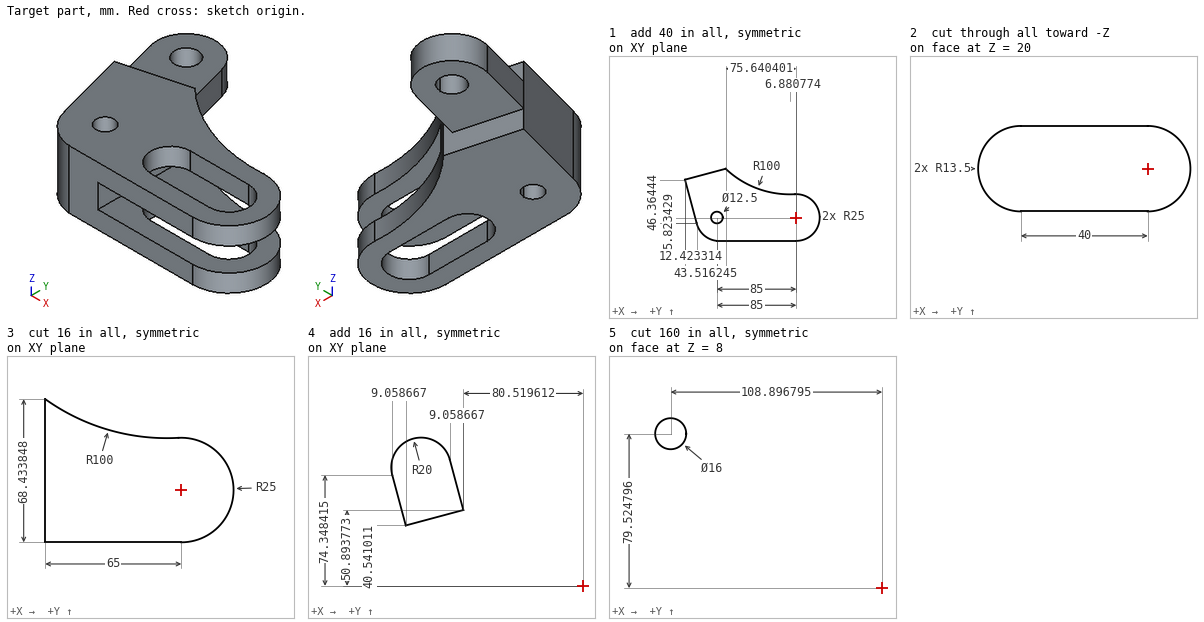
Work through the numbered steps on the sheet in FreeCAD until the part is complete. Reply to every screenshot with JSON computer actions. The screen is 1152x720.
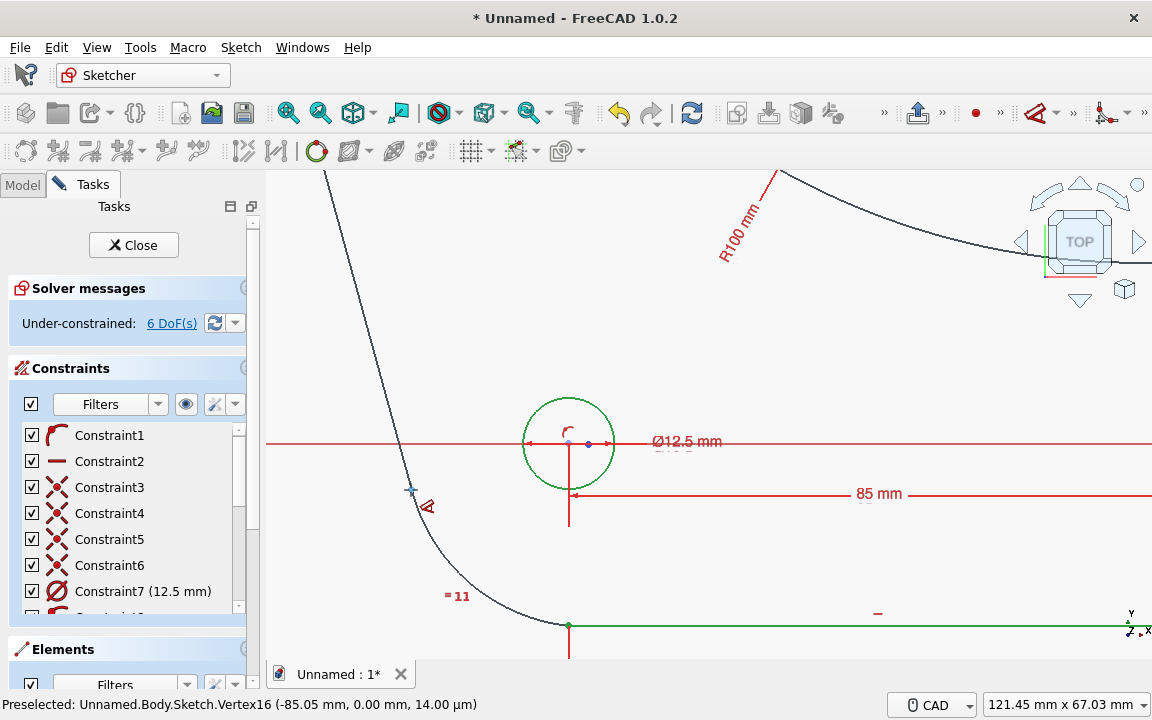
{"action": "left_click", "coordinate": [412, 489]}
{"action": "left_click", "coordinate": [378, 466]}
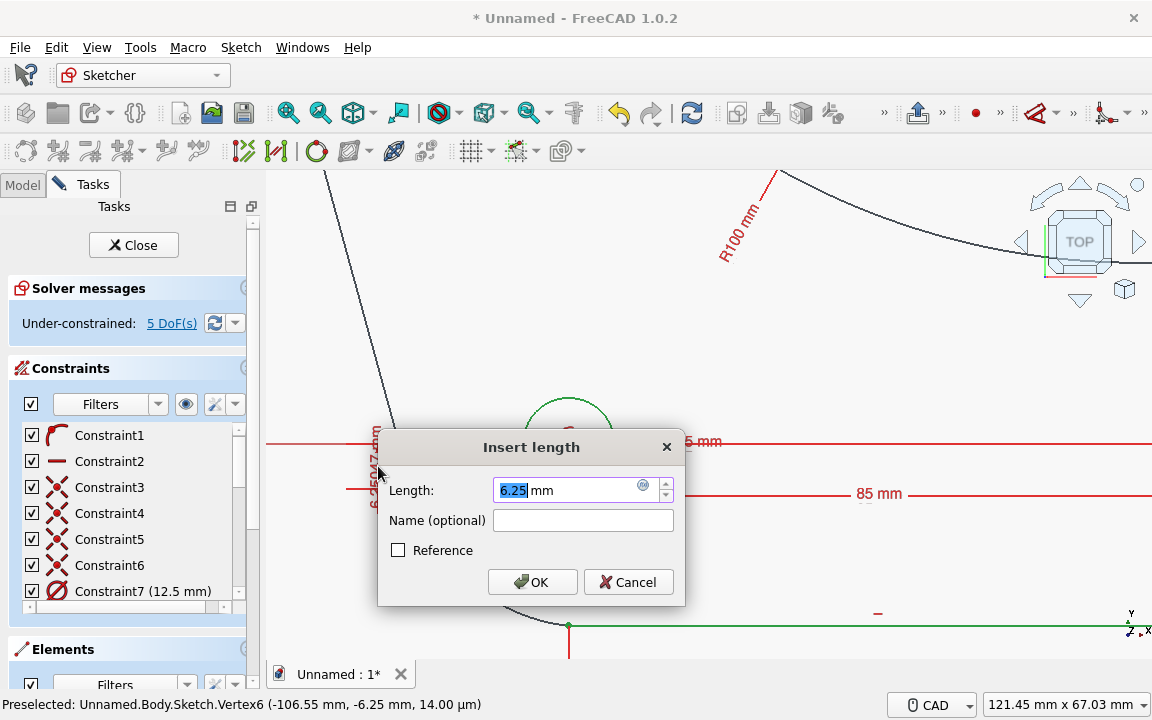
{"action": "type", "text": "5.823429"}
{"action": "key", "text": "Return"}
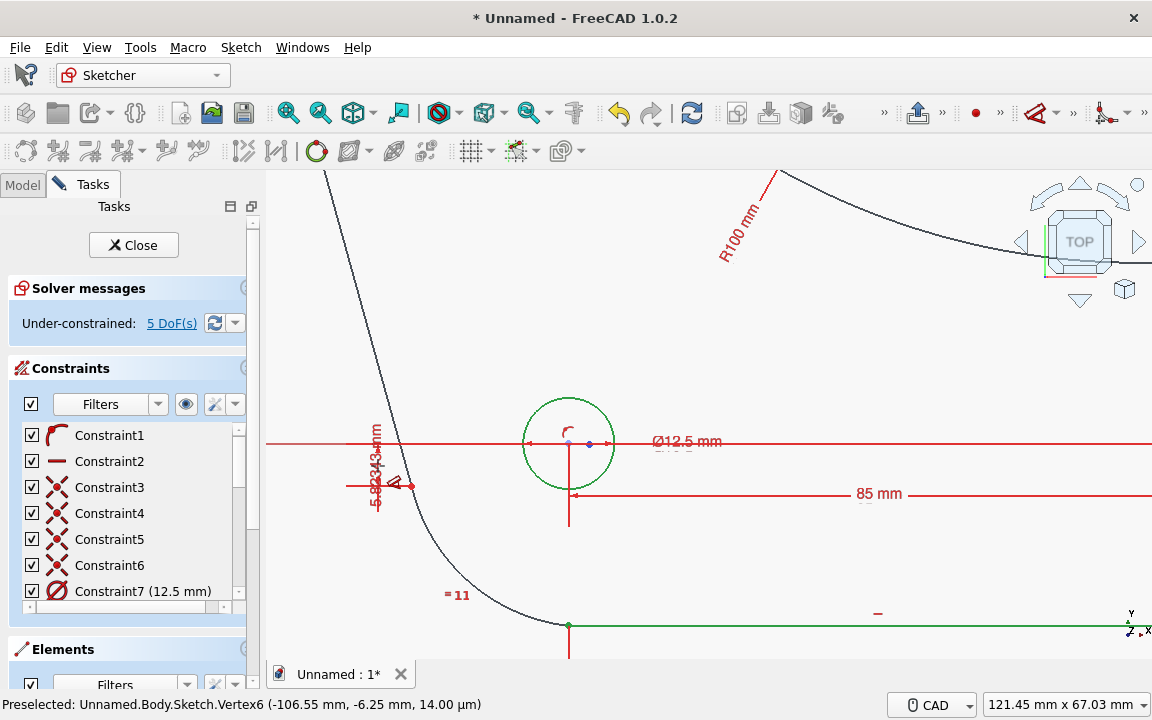
{"action": "left_click", "coordinate": [347, 251]}
{"action": "left_click", "coordinate": [446, 342]}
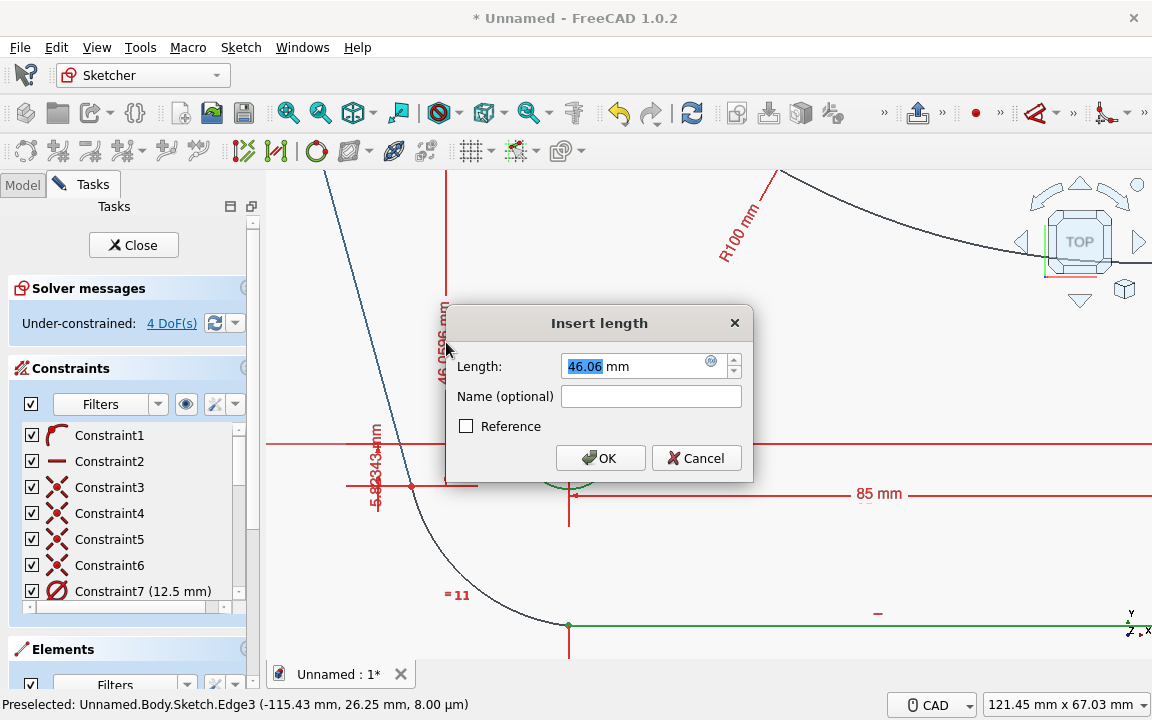
{"action": "type", "text": "46.36444"}
{"action": "key", "text": "Return"}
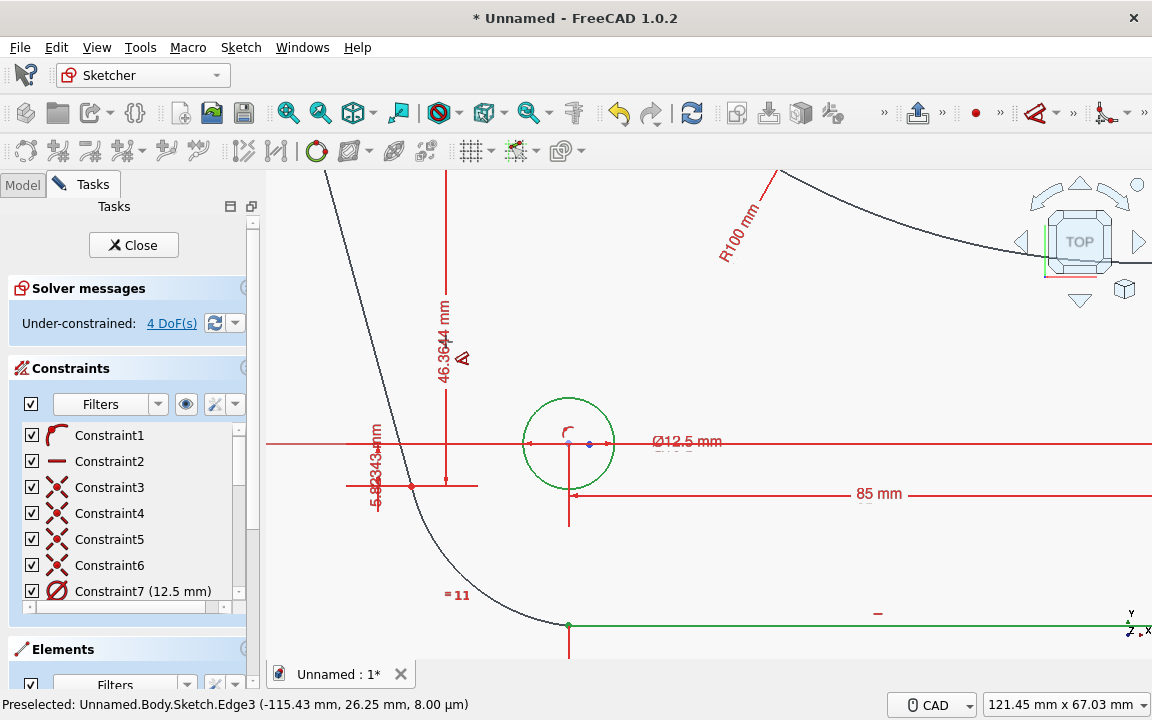
{"action": "scroll", "coordinate": [473, 472], "scroll_direction": "down", "scroll_amount": 4}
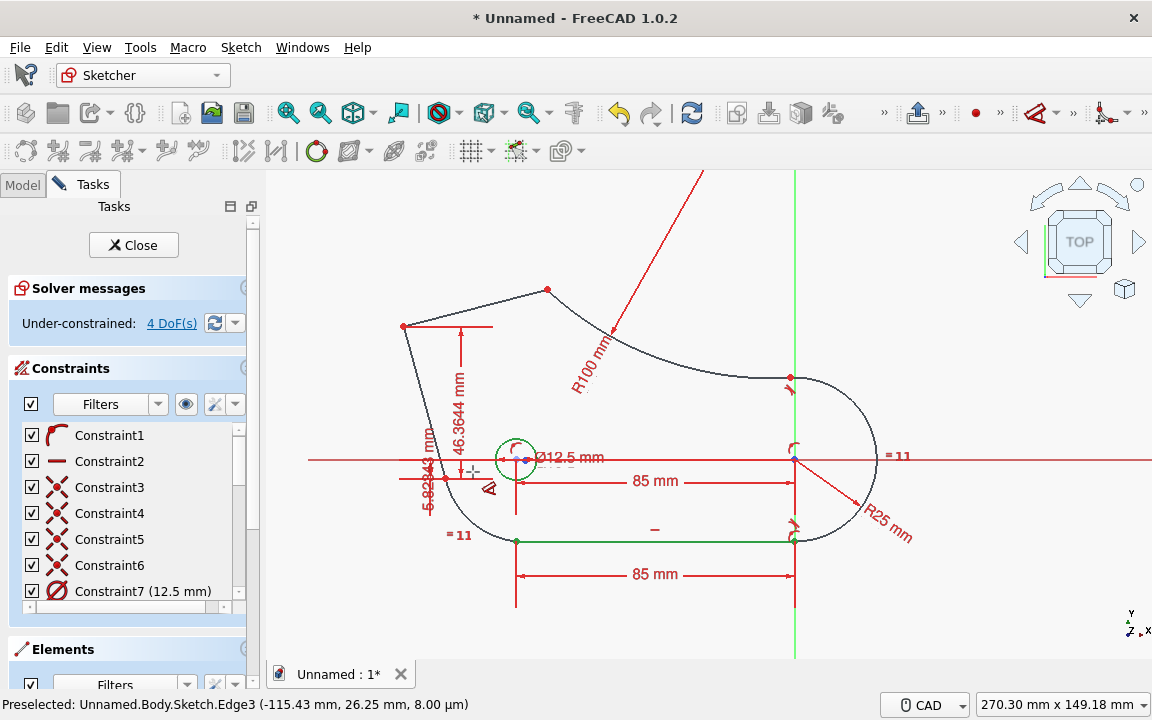
{"action": "scroll", "coordinate": [641, 631], "scroll_direction": "down", "scroll_amount": 2}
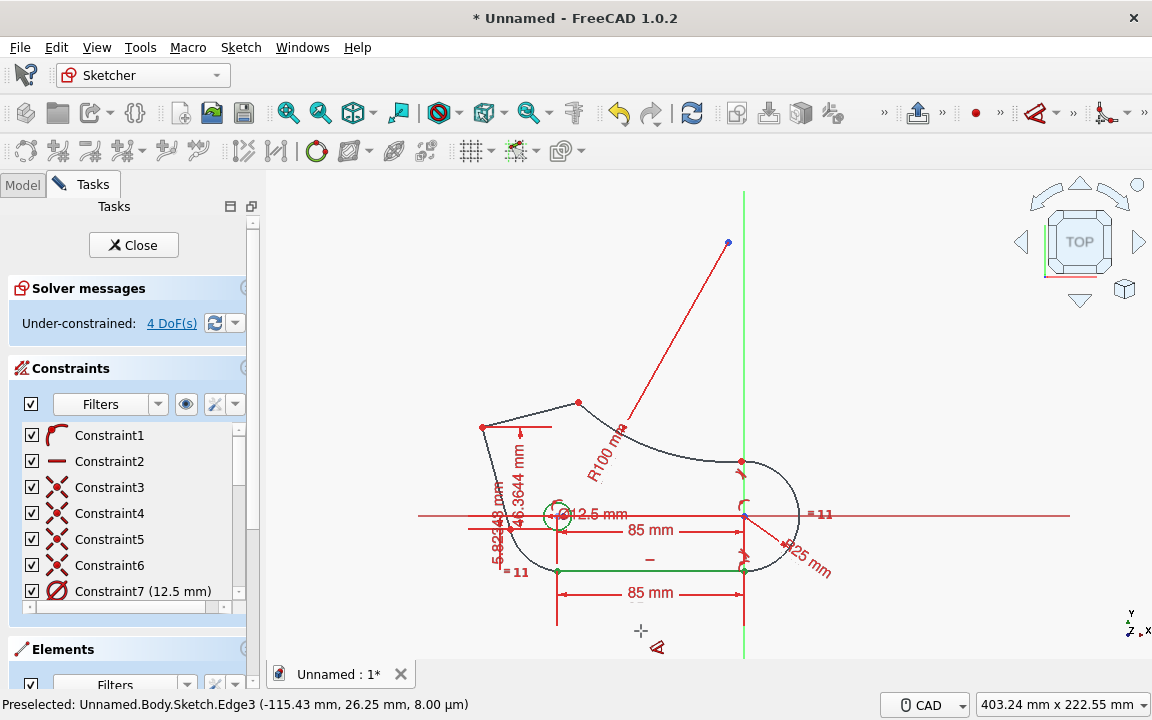
{"action": "scroll", "coordinate": [728, 242], "scroll_direction": "up", "scroll_amount": 5}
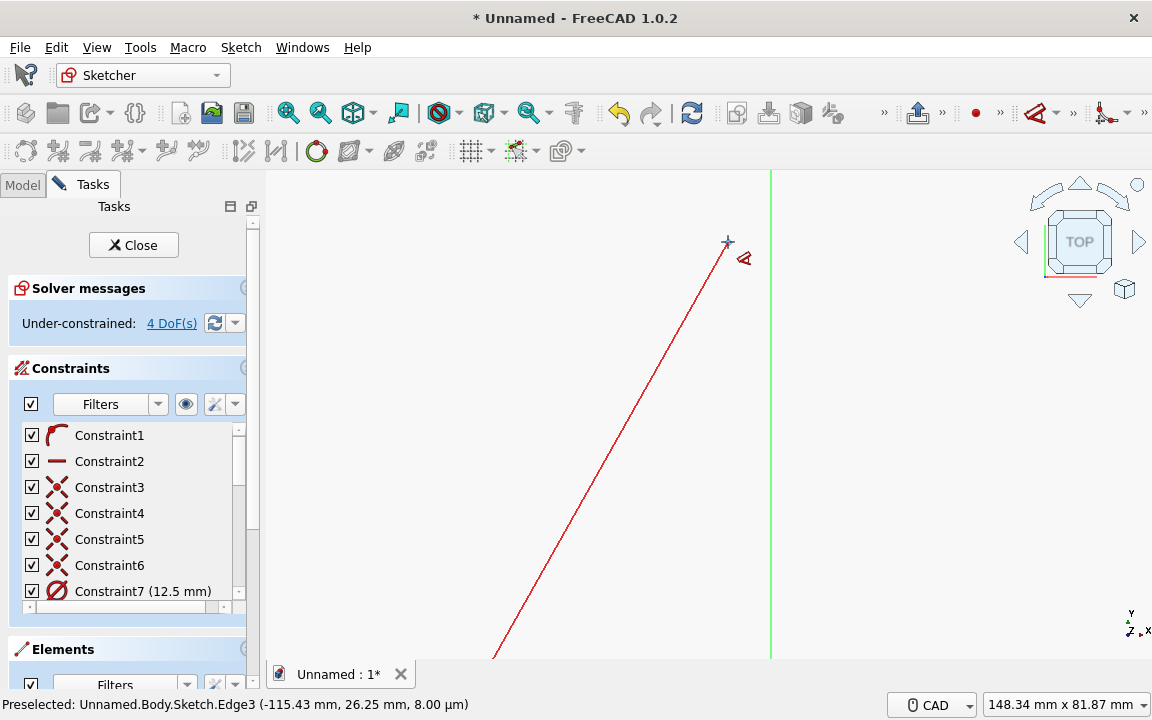
{"action": "left_click", "coordinate": [728, 242]}
{"action": "left_click", "coordinate": [750, 208]}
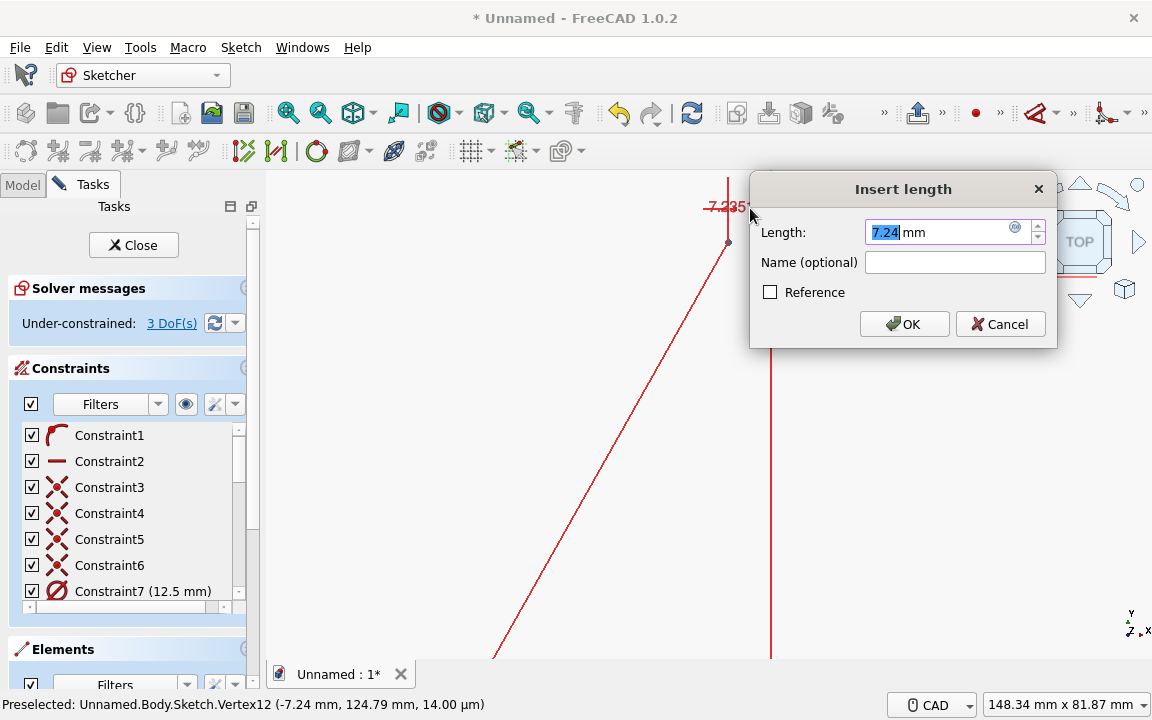
{"action": "type", "text": "6.880774"}
{"action": "key", "text": "Return"}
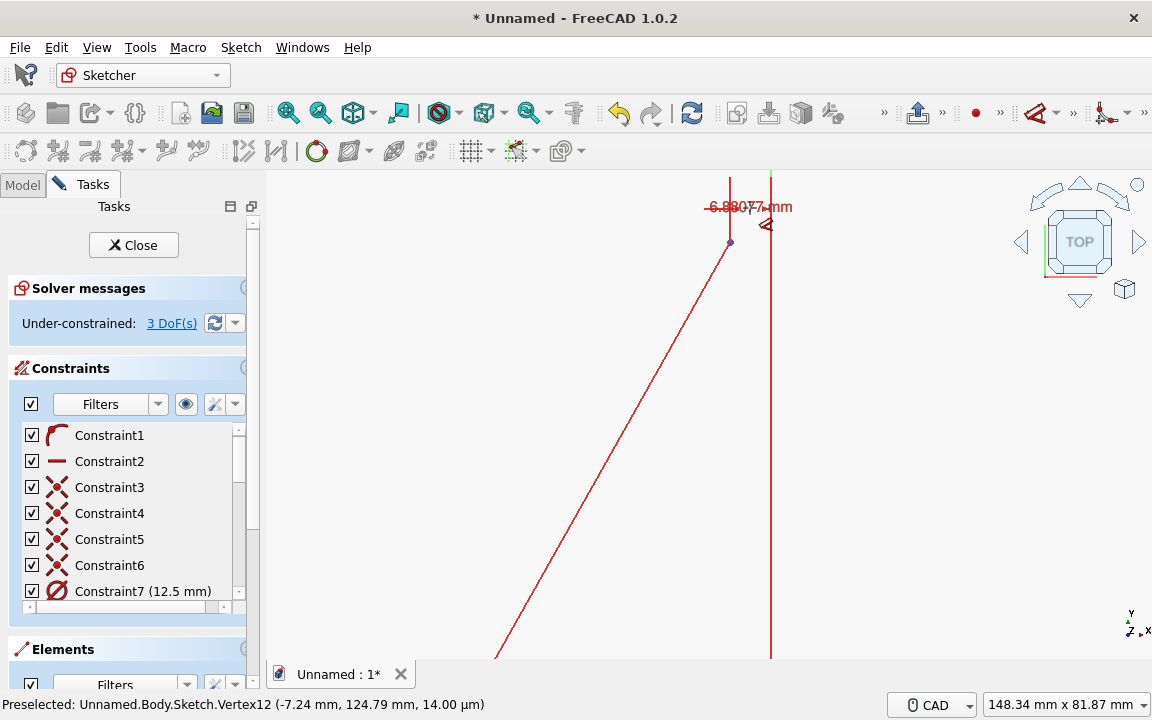
{"action": "scroll", "coordinate": [728, 198], "scroll_direction": "down", "scroll_amount": 5}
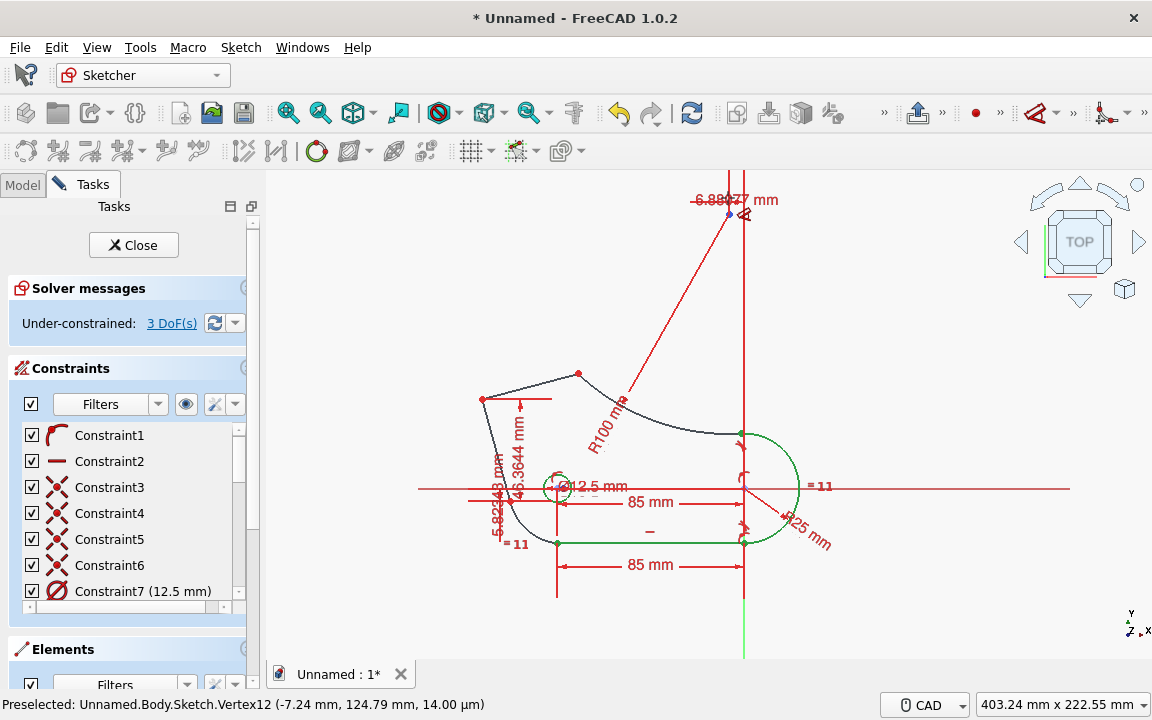
{"action": "scroll", "coordinate": [641, 548], "scroll_direction": "up", "scroll_amount": 2}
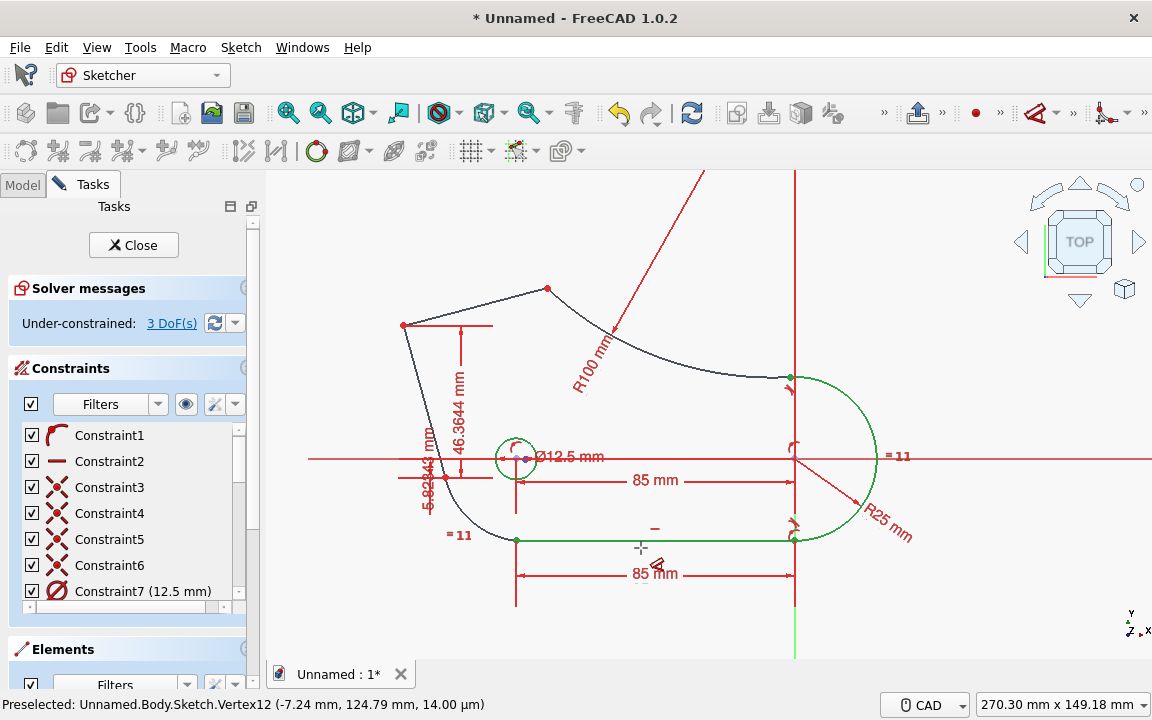
{"action": "left_click", "coordinate": [547, 288]}
{"action": "left_click", "coordinate": [671, 254]}